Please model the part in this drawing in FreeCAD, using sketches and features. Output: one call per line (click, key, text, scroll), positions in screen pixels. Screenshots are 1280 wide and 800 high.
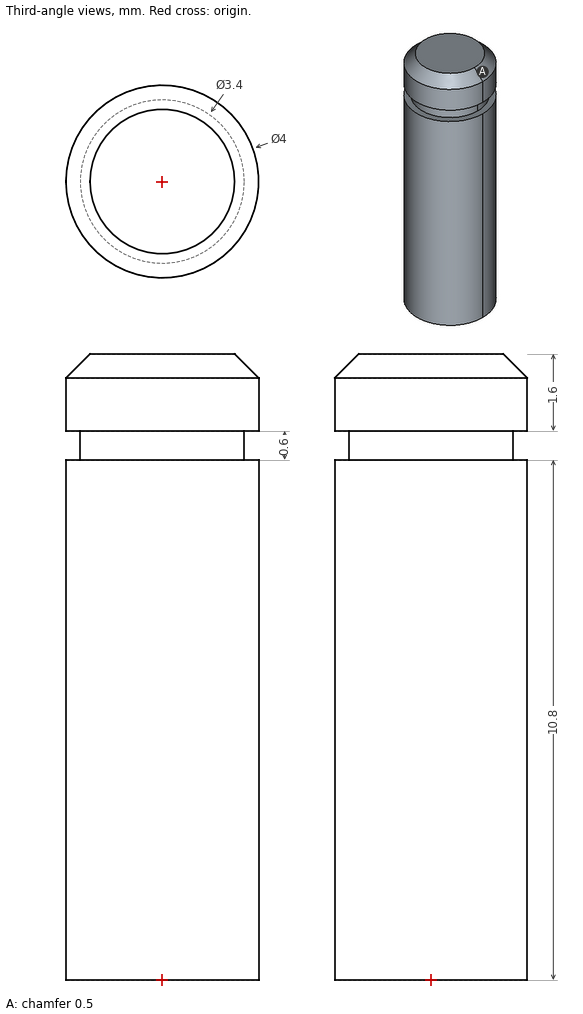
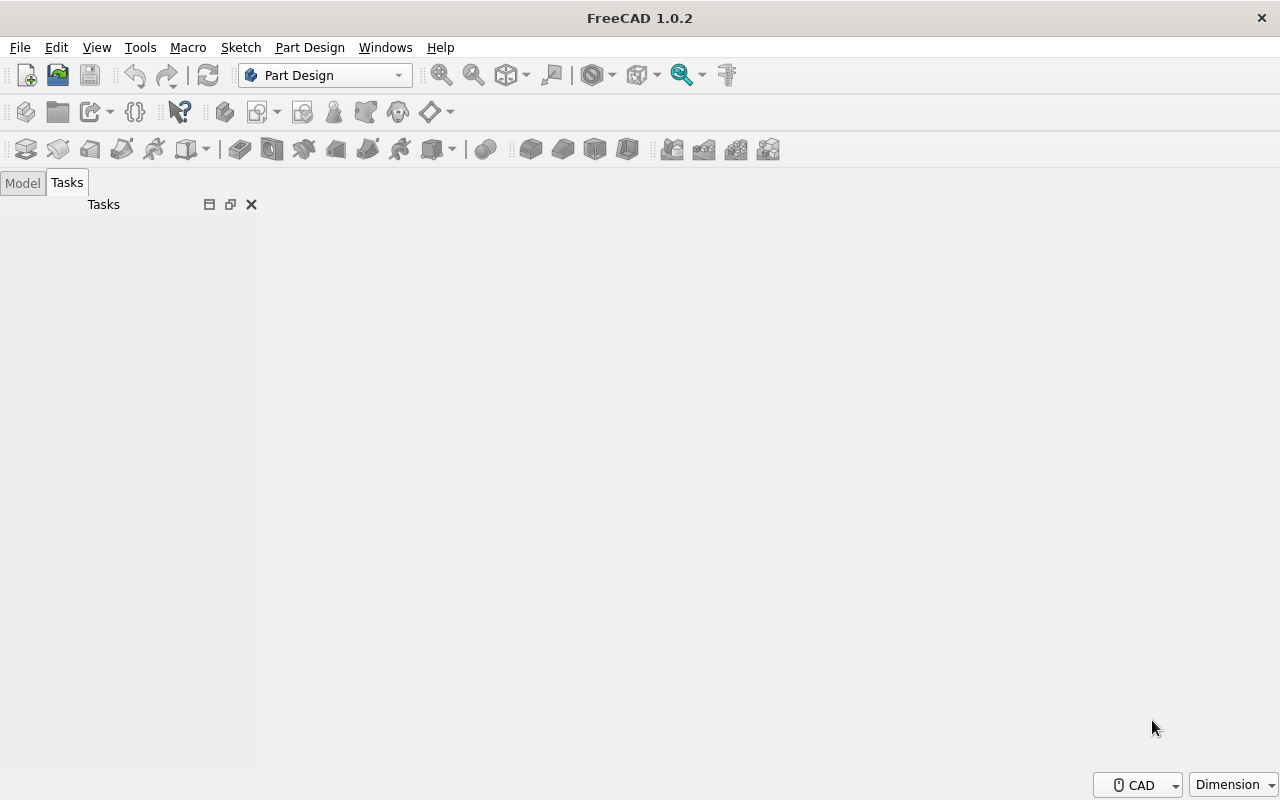
key(ctrl+n)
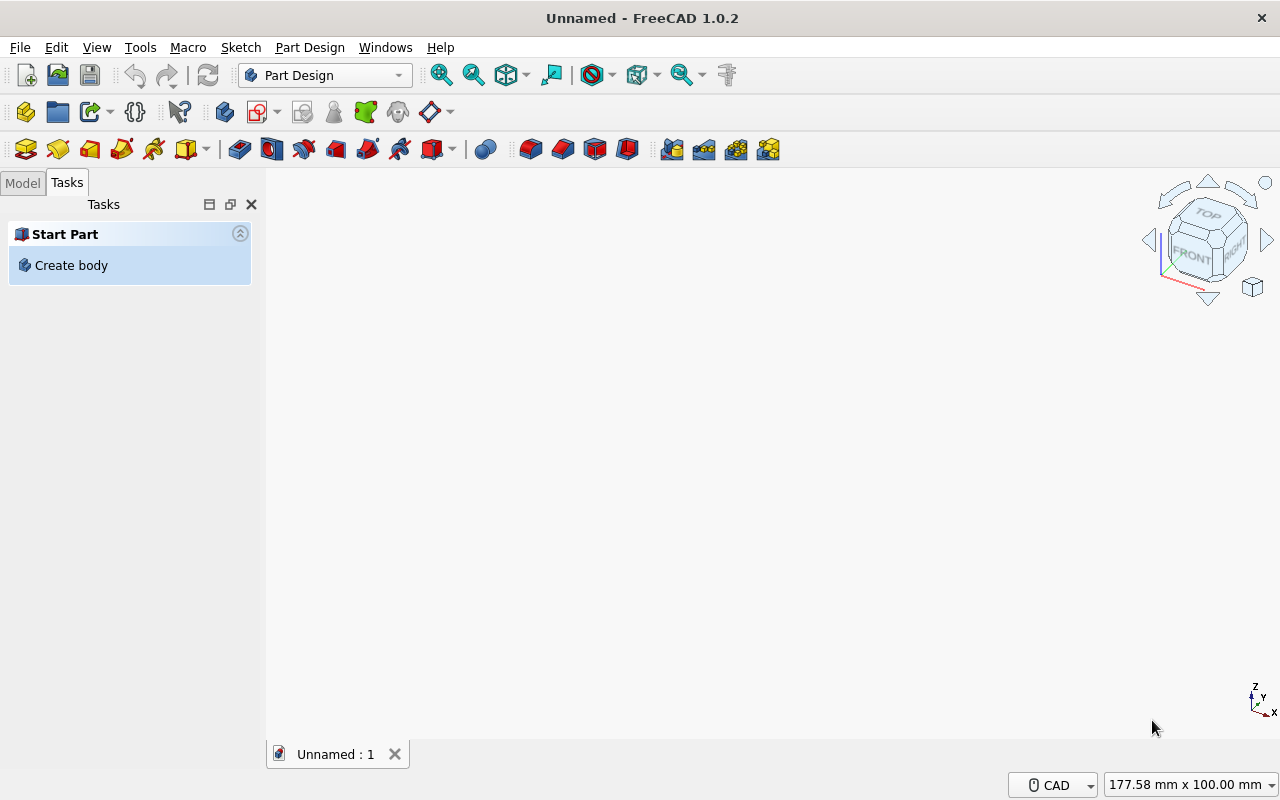
click(258, 112)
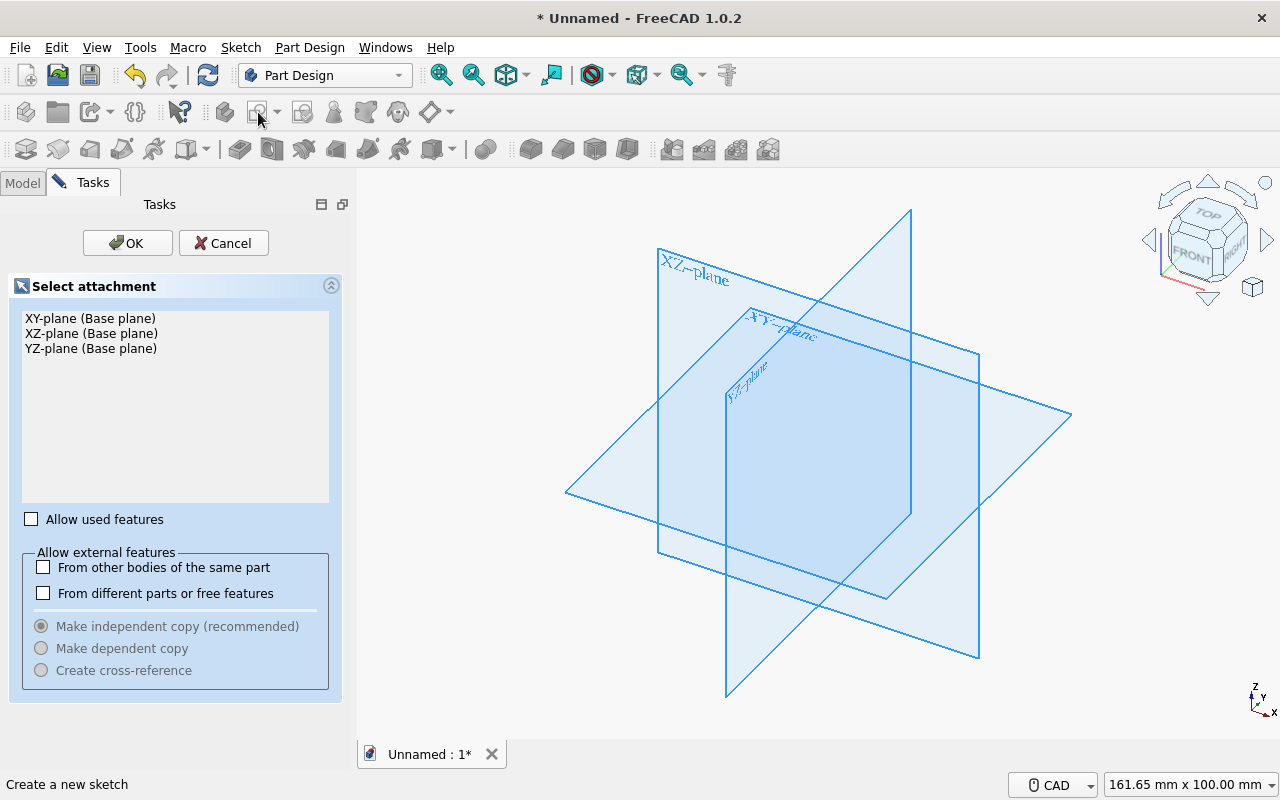
click(82, 318)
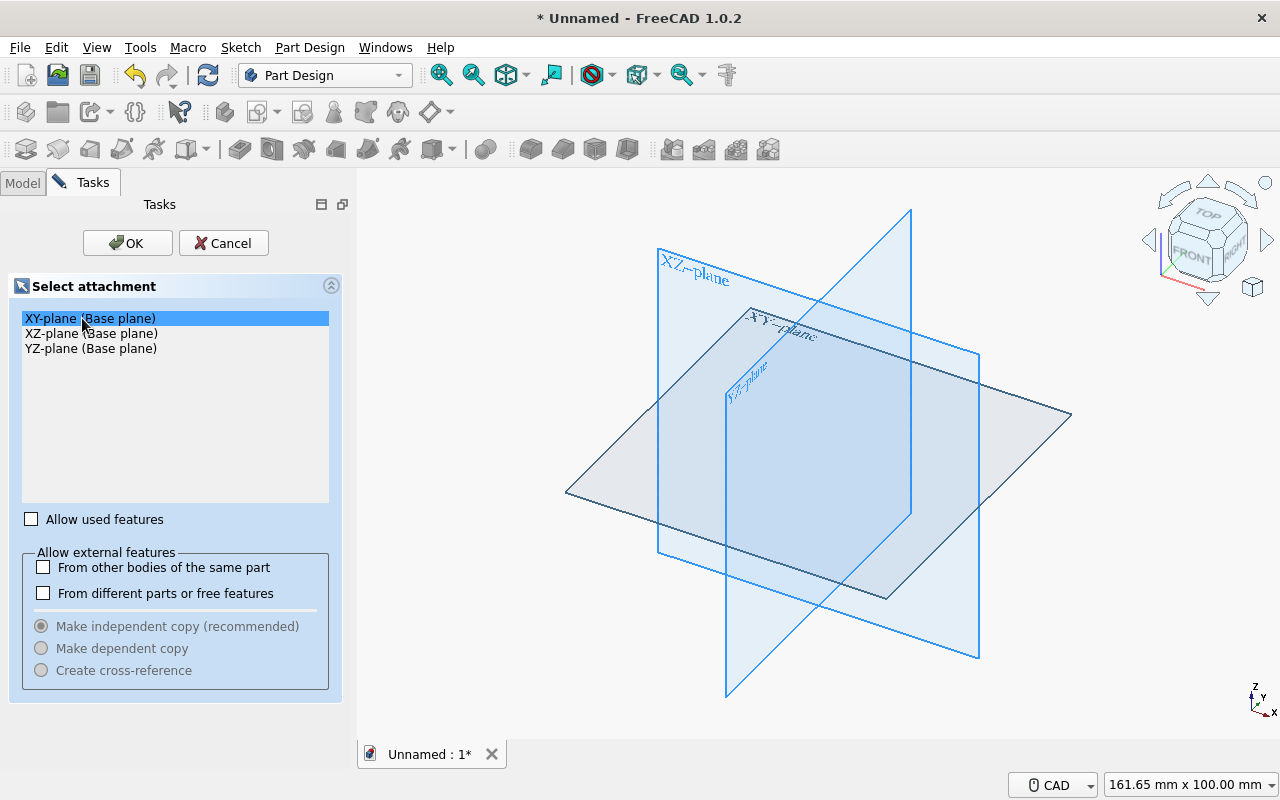
click(128, 243)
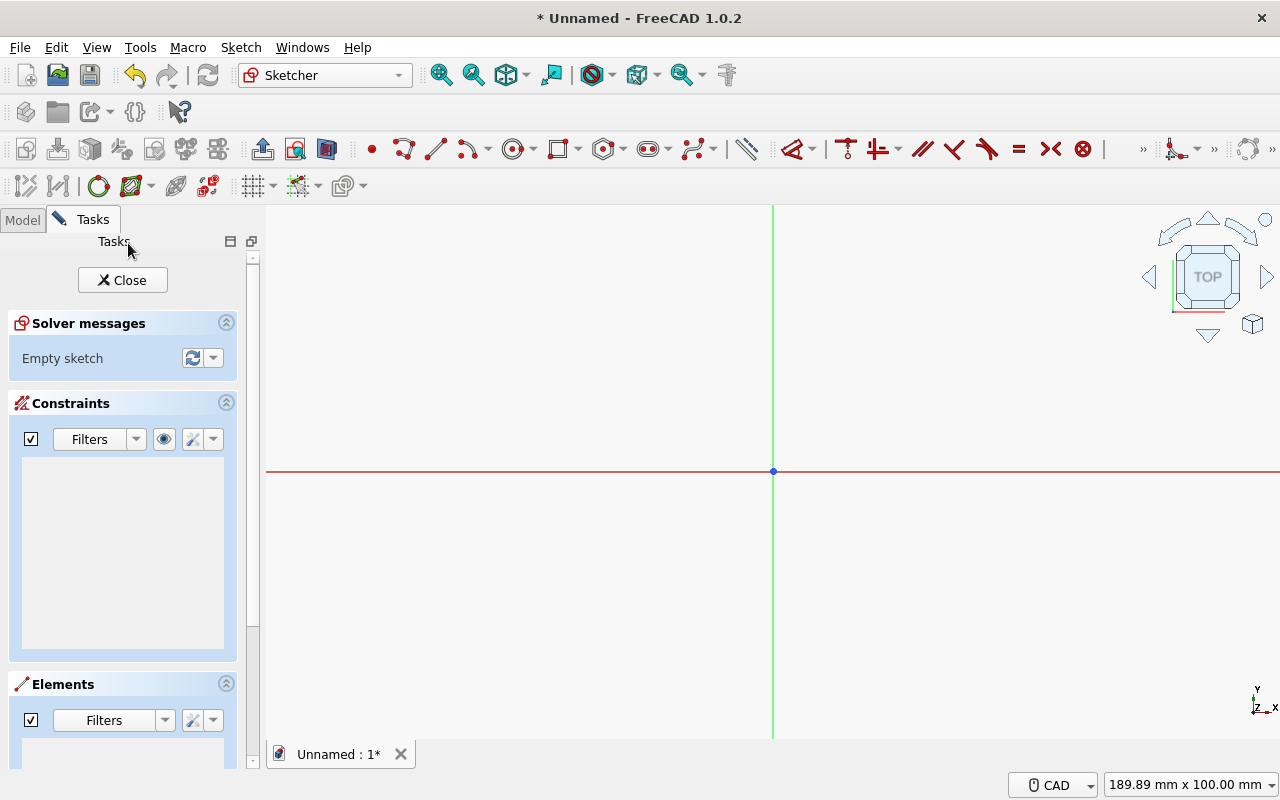
scroll(777, 472, up, 14)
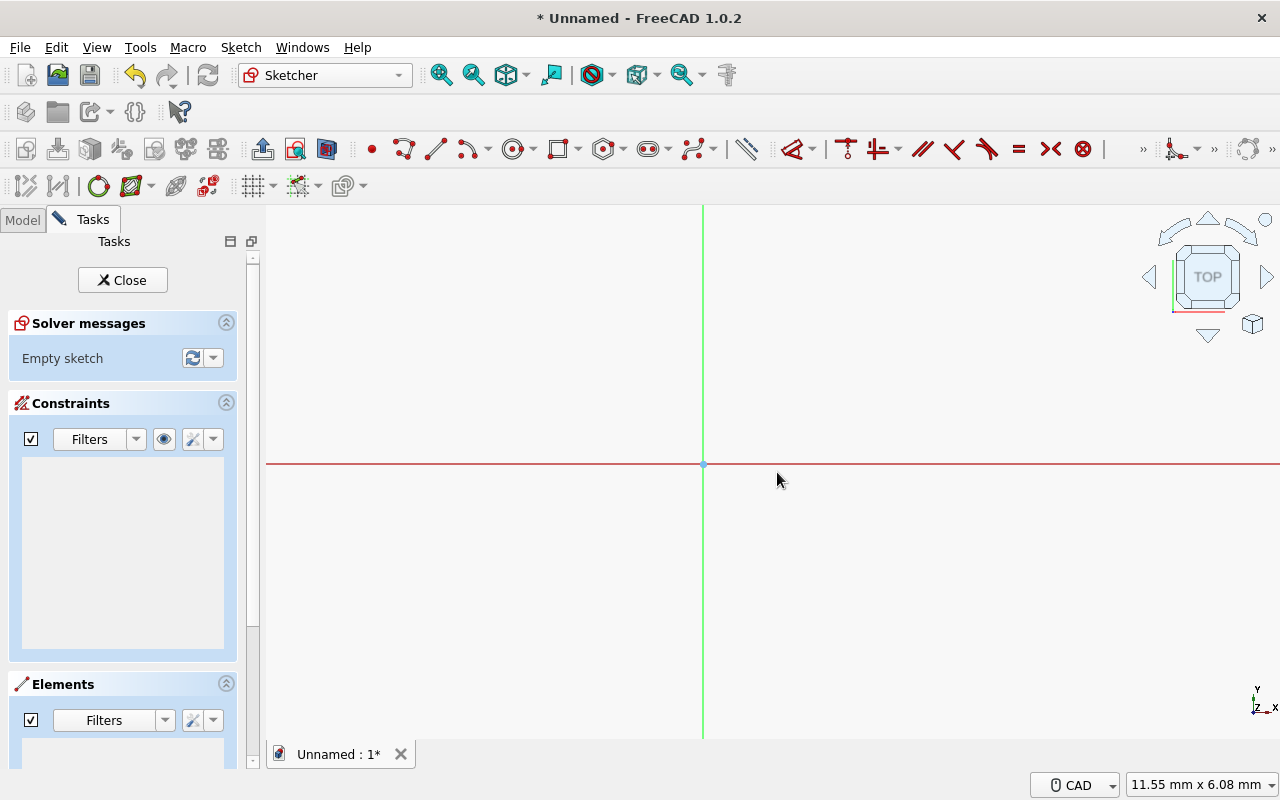
key(g)
key(c)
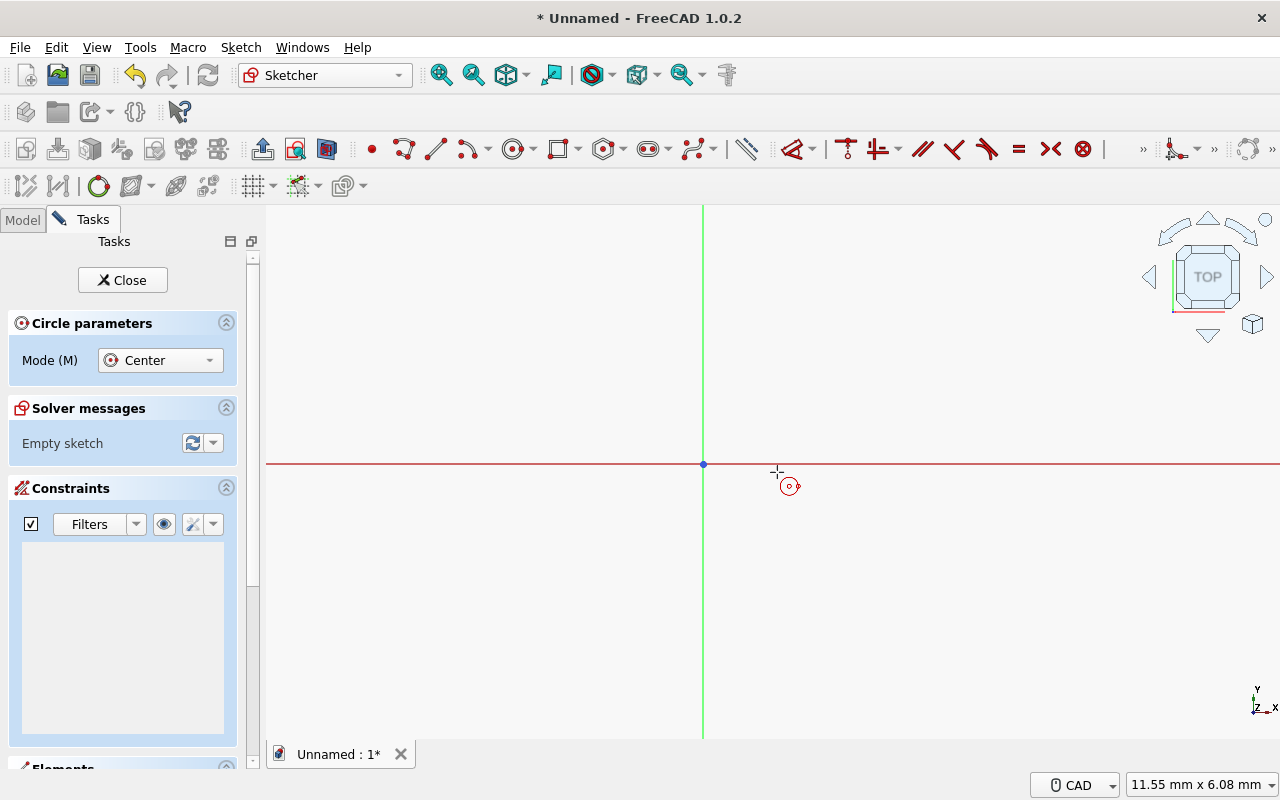
click(703, 464)
click(828, 340)
key(Escape)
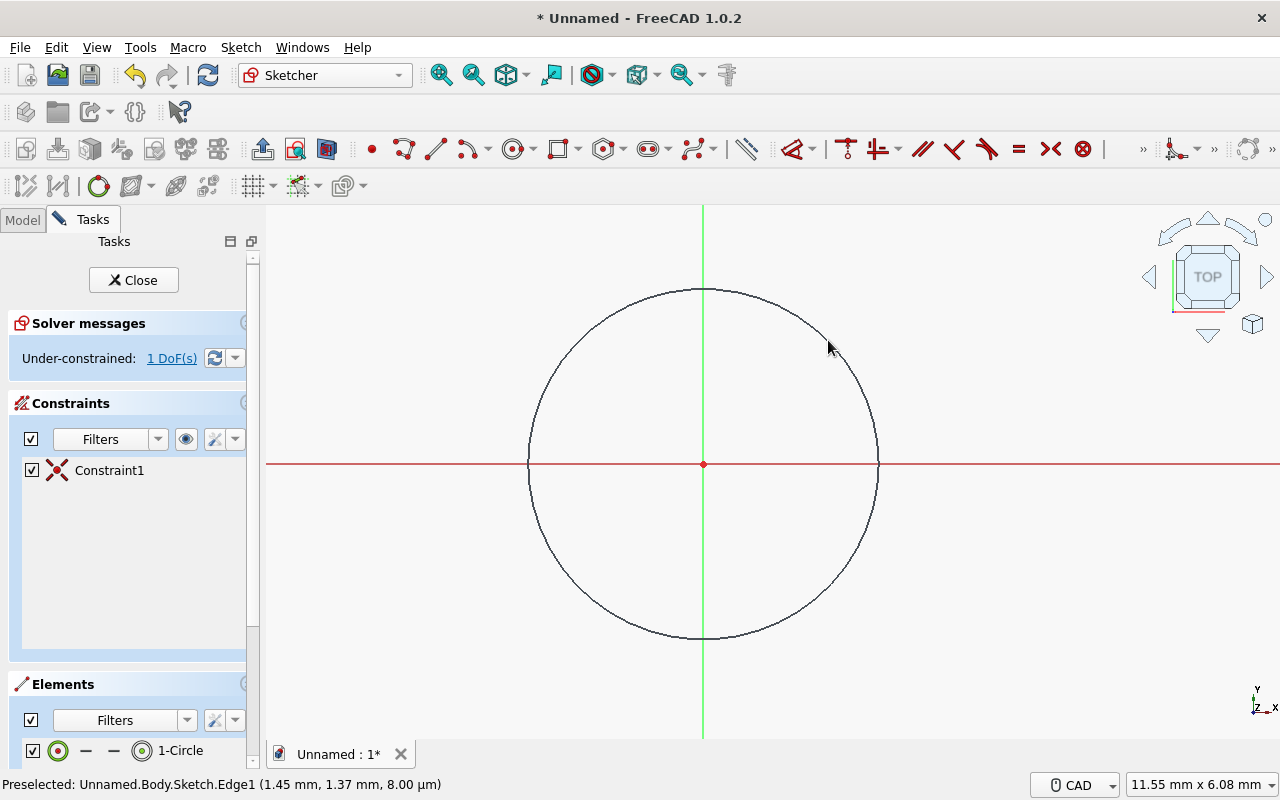
click(792, 150)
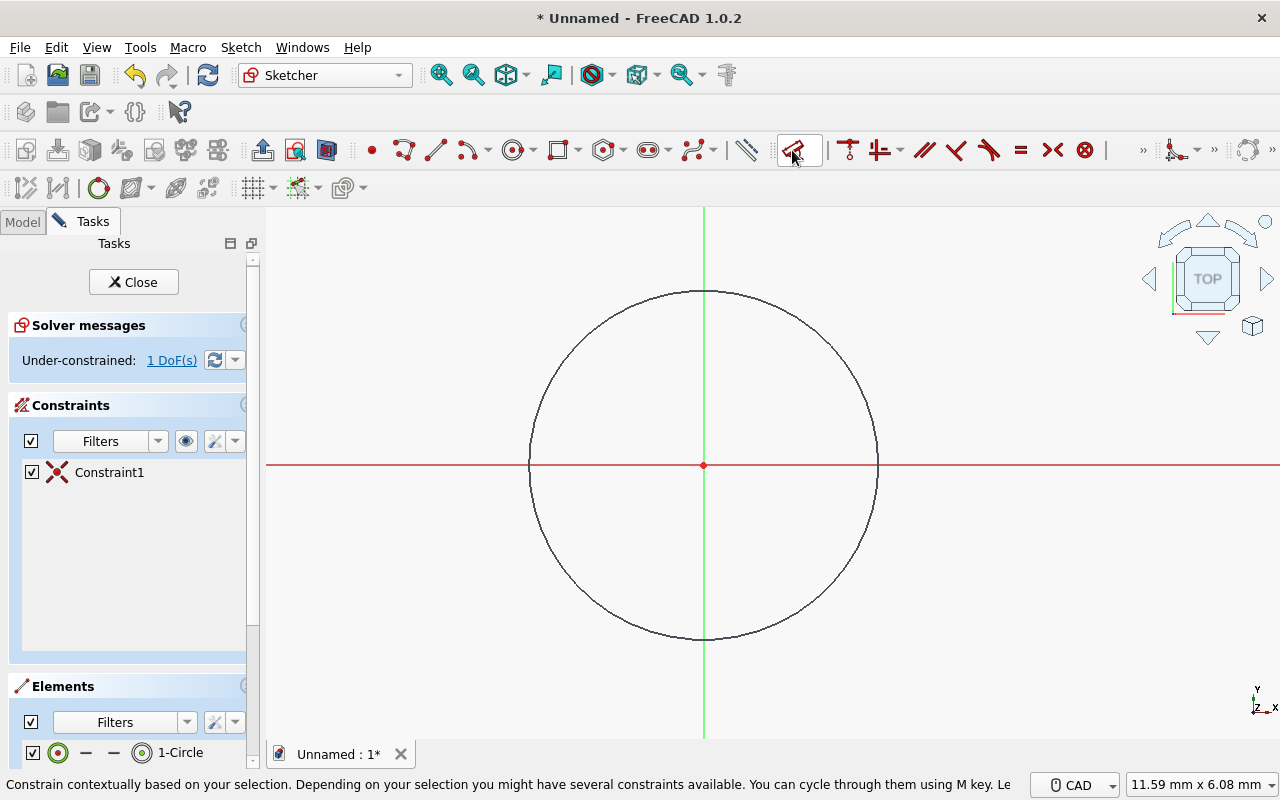
click(827, 341)
click(850, 318)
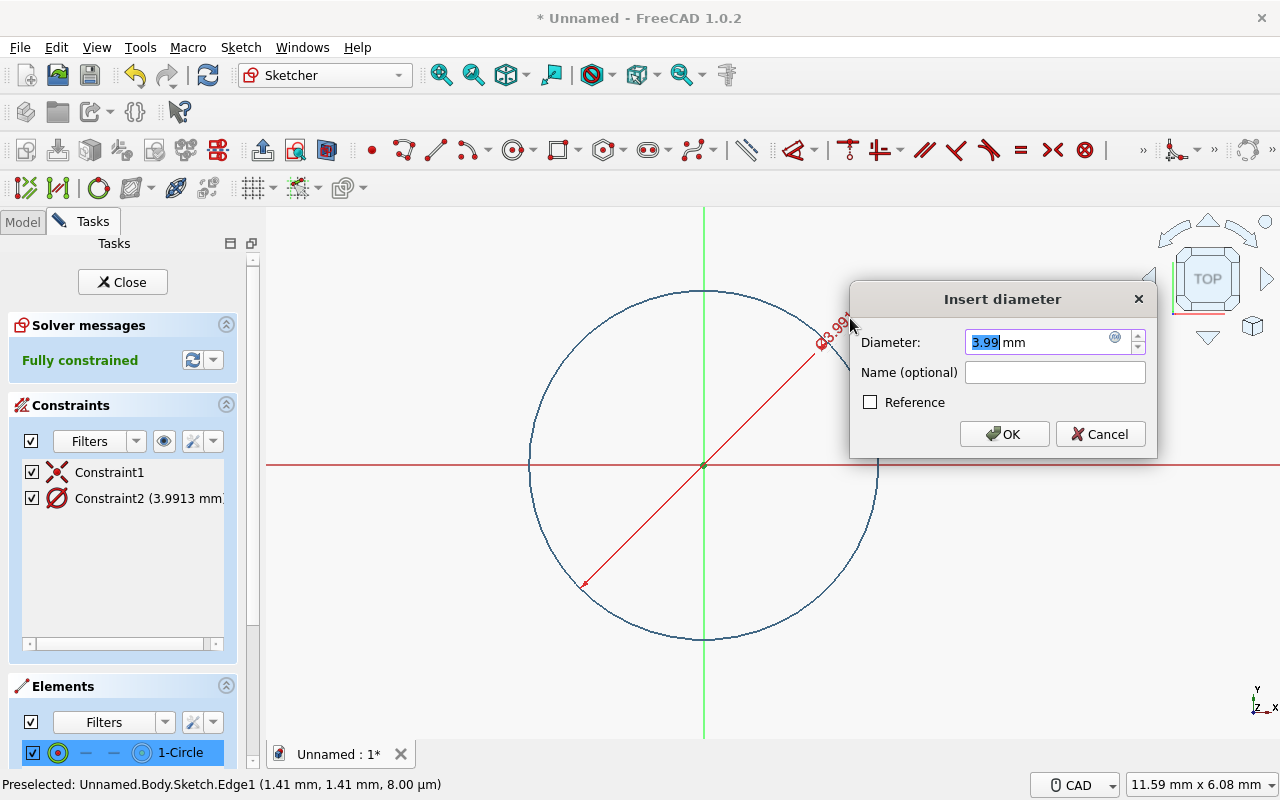
text(4)
key(Return)
key(Escape)